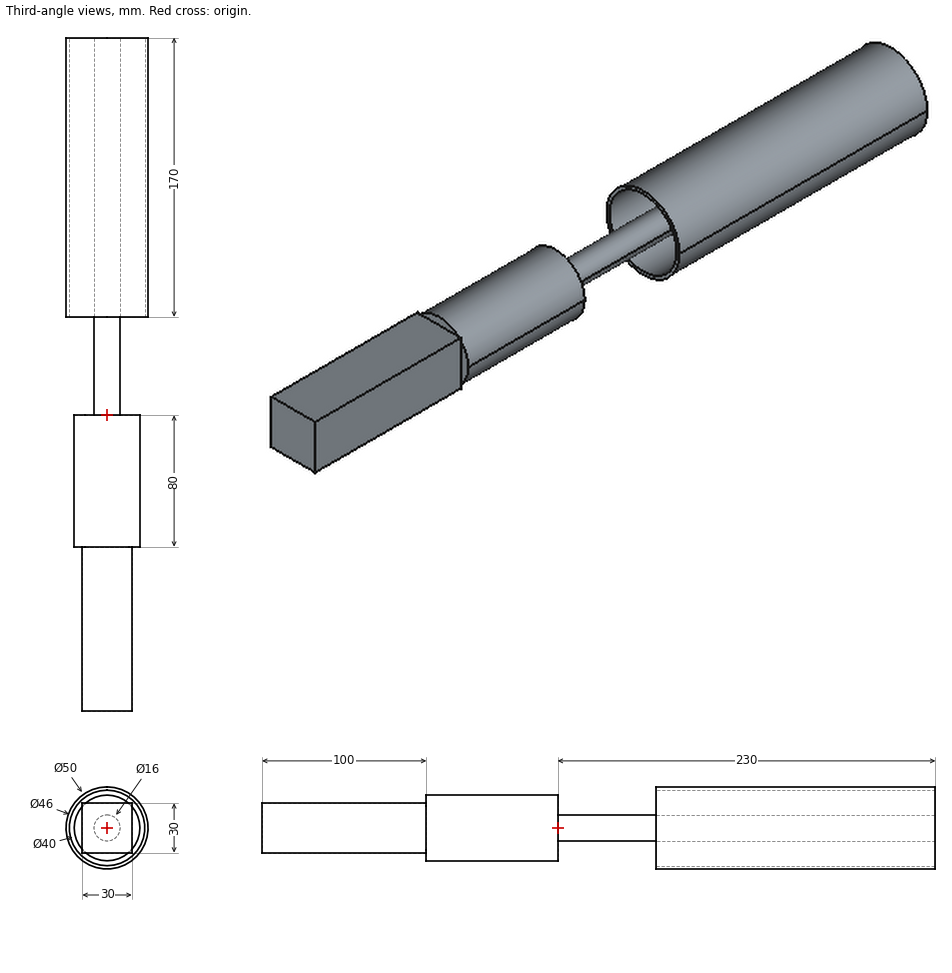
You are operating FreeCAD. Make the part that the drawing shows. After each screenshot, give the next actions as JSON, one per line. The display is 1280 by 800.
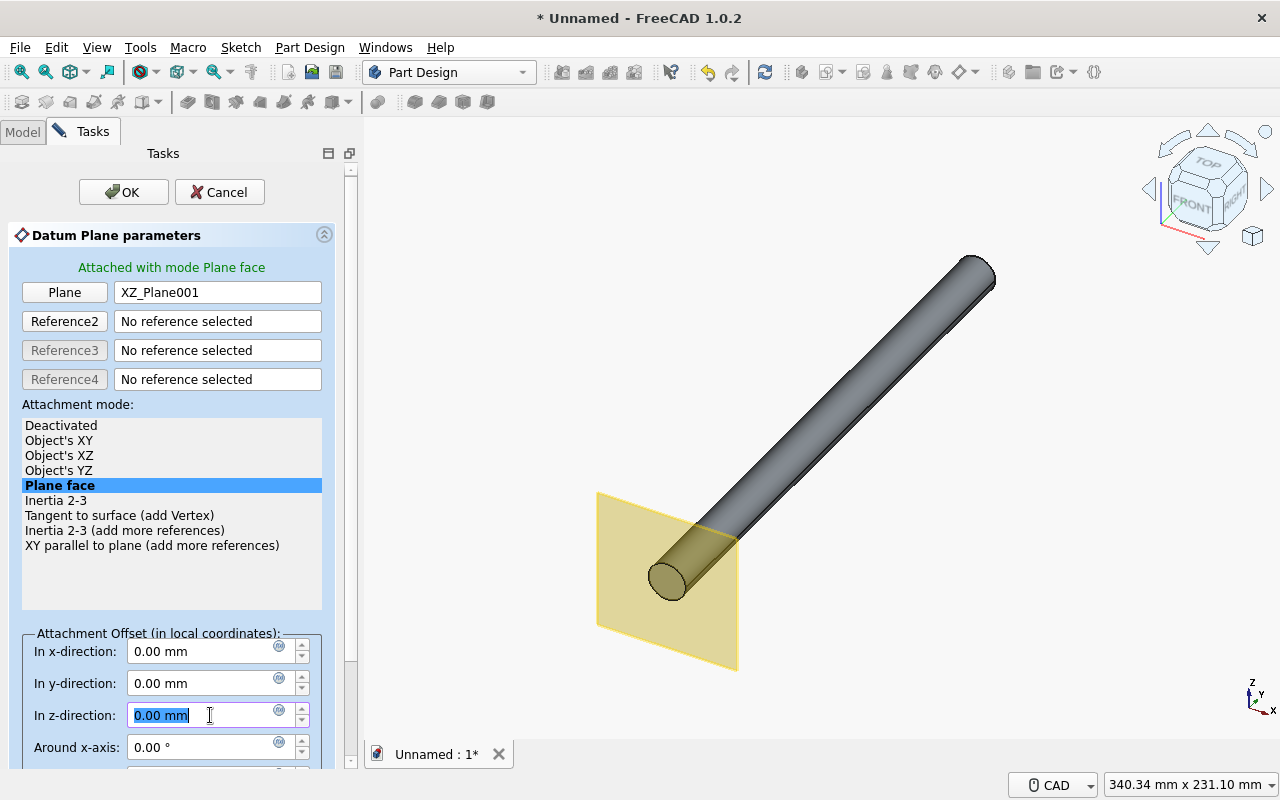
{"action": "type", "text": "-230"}
{"action": "key", "text": "Tab"}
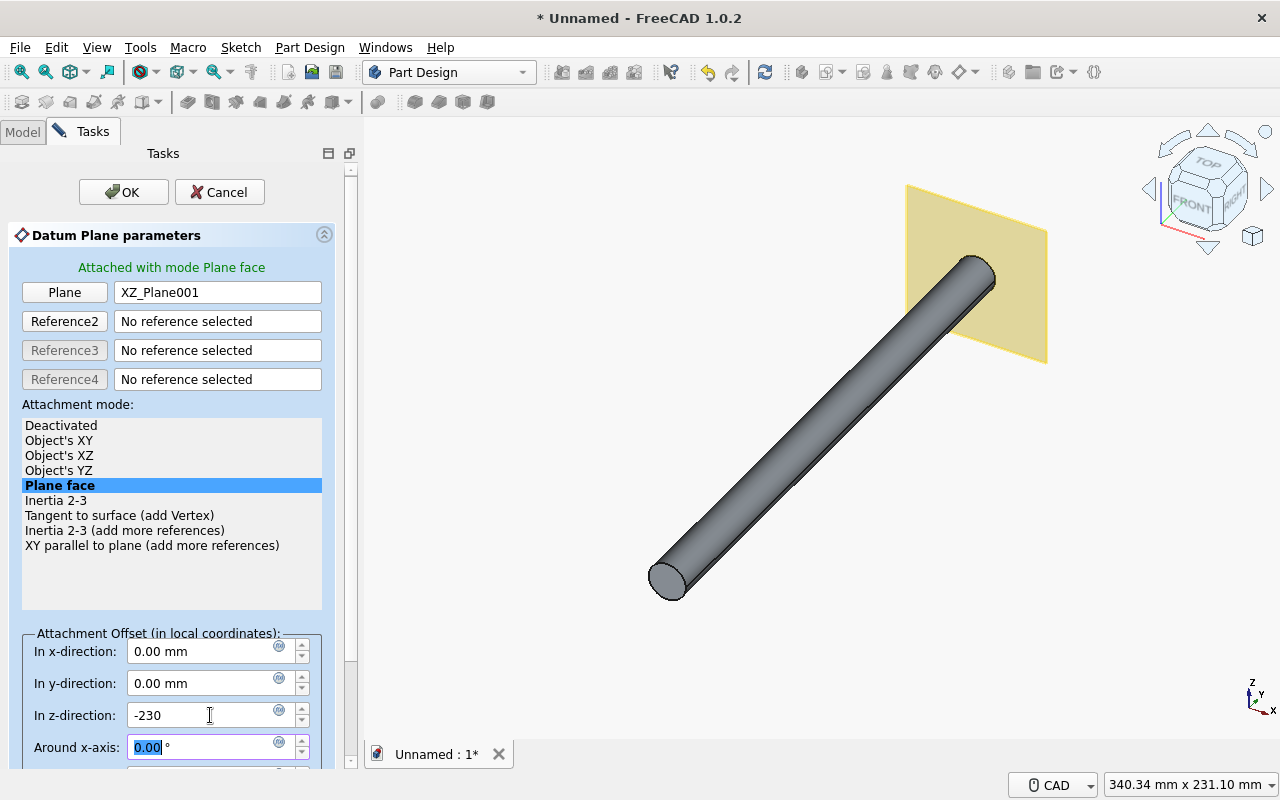
{"action": "left_click", "coordinate": [124, 192]}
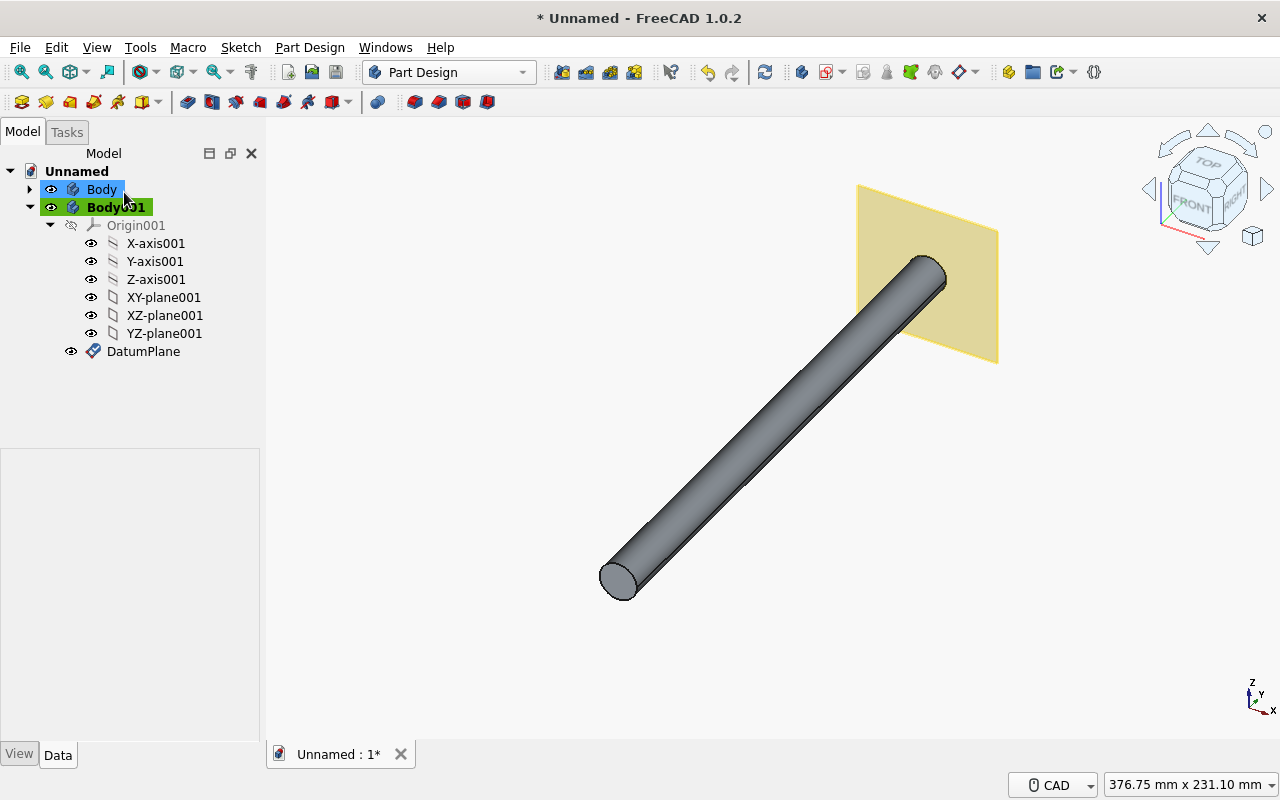
{"action": "left_click", "coordinate": [116, 351]}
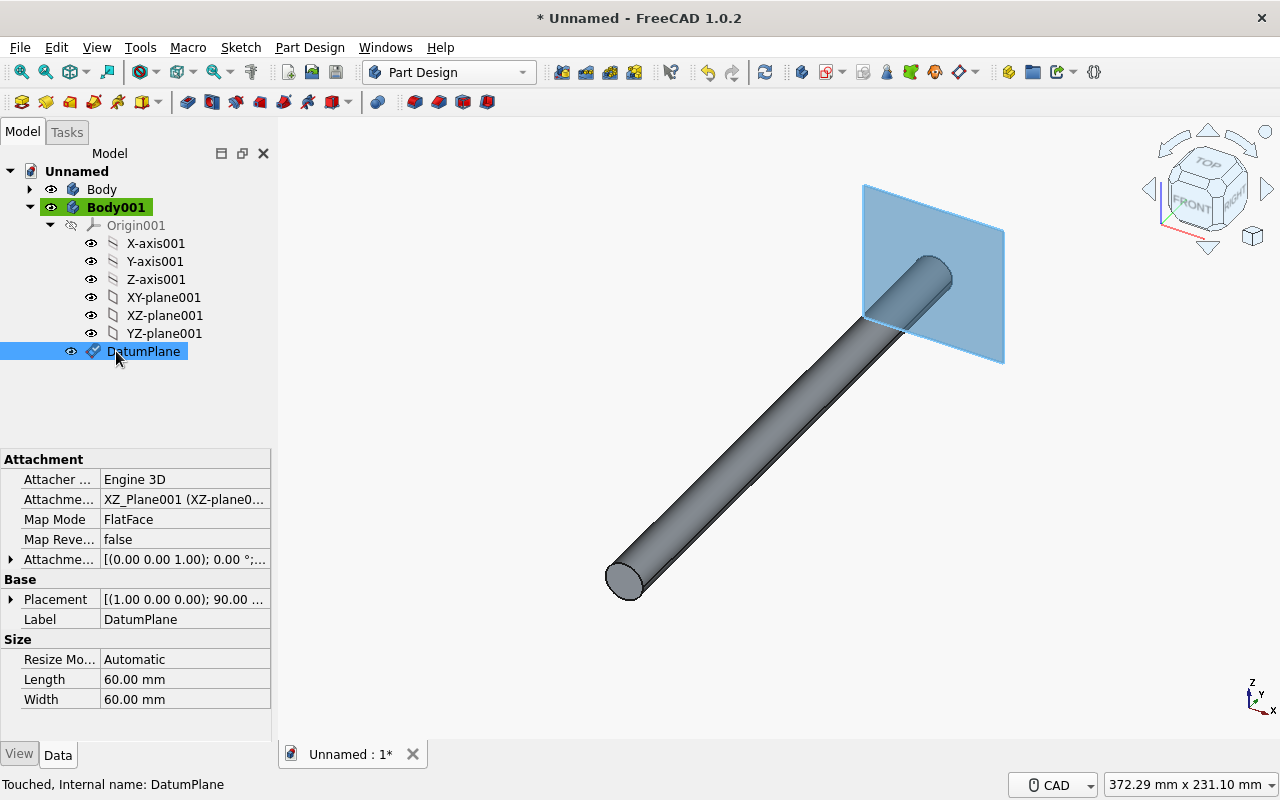
{"action": "left_click", "coordinate": [826, 72]}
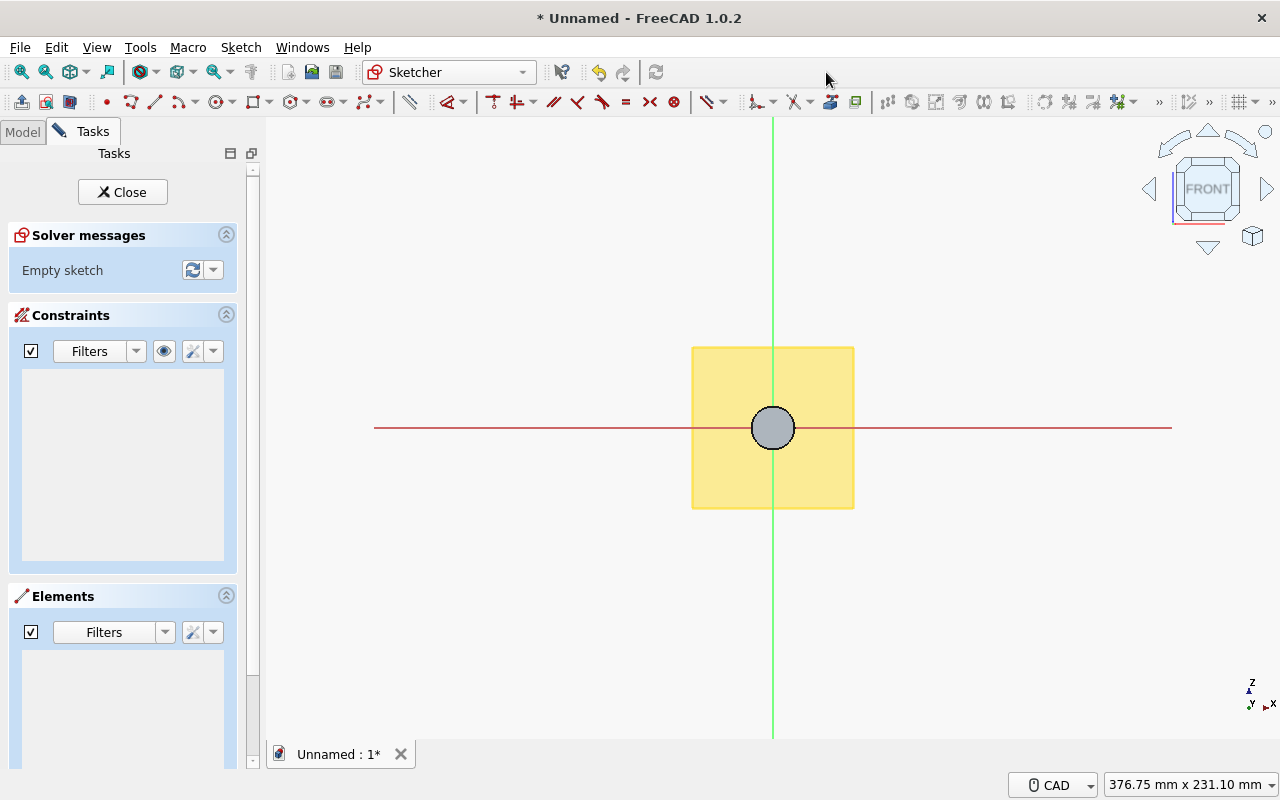
{"action": "scroll", "coordinate": [813, 428], "scroll_direction": "up", "scroll_amount": 5}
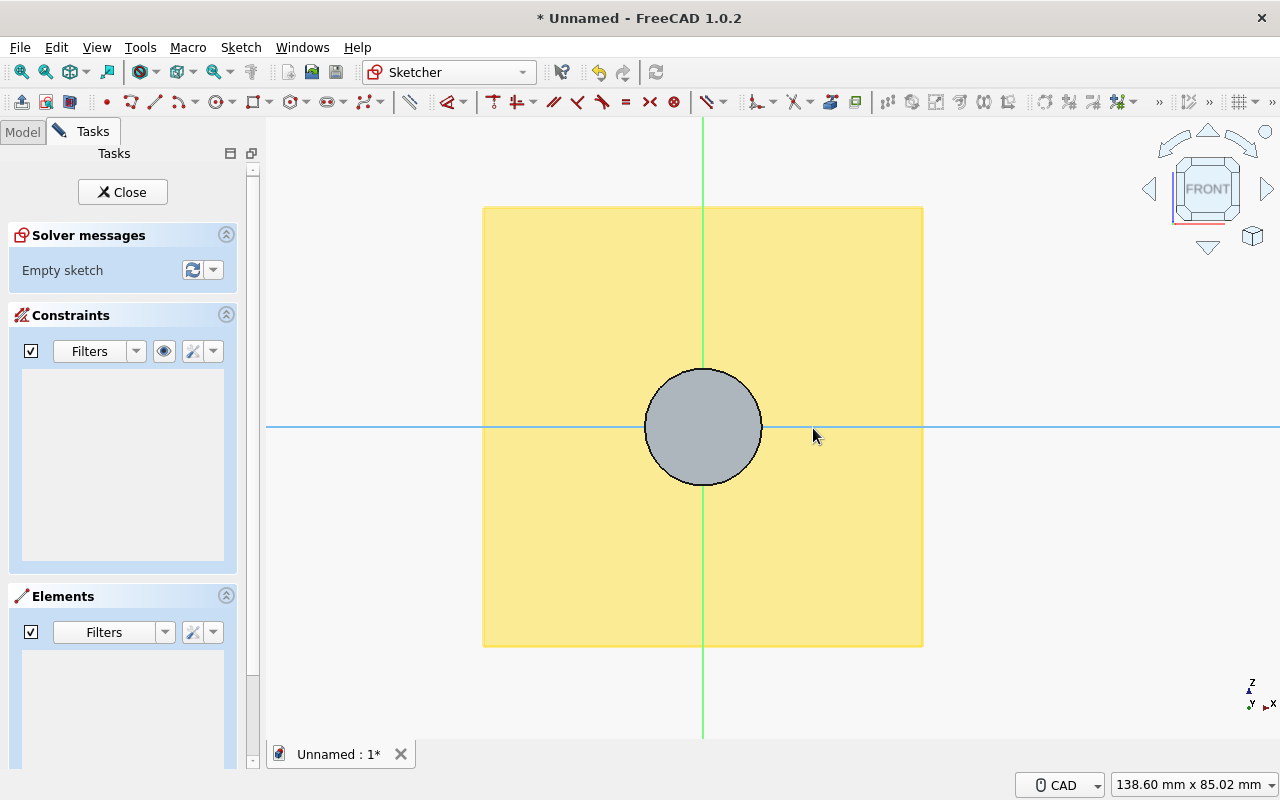
{"action": "left_click", "coordinate": [216, 102]}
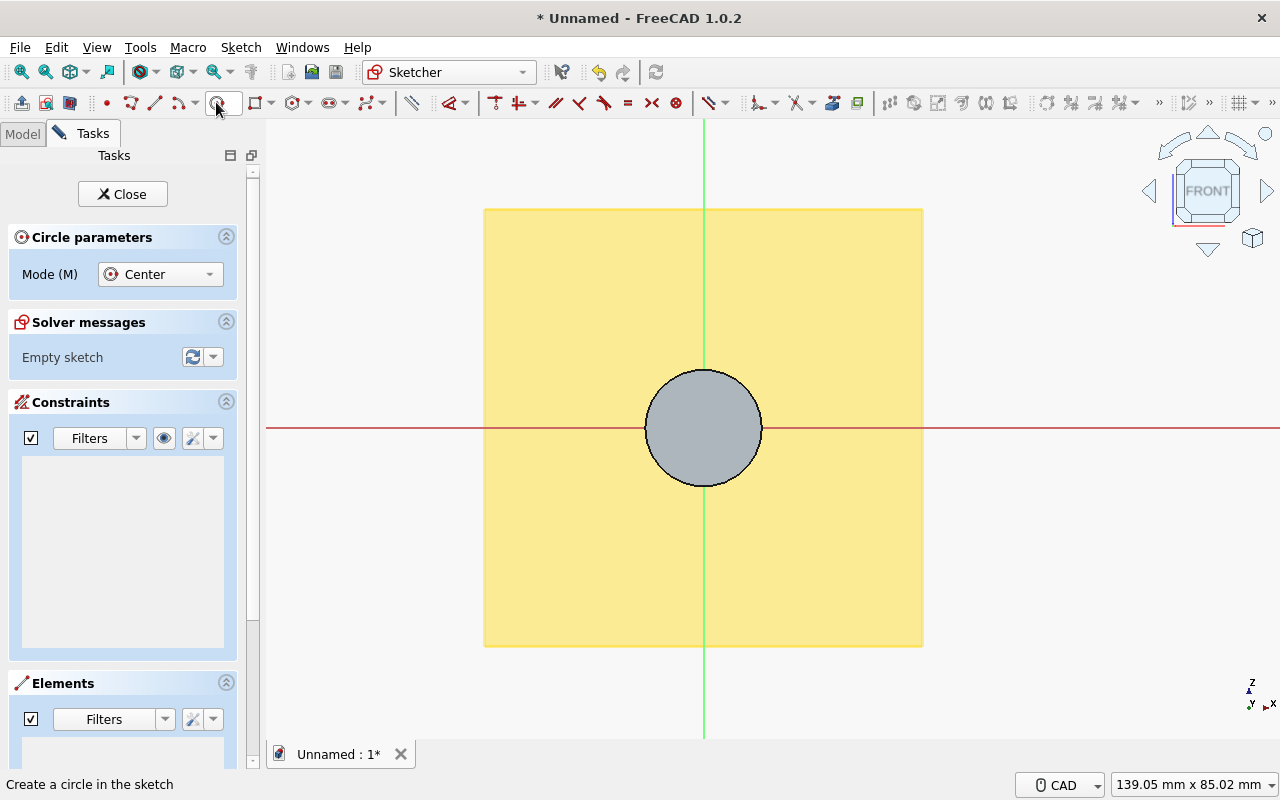
{"action": "left_click", "coordinate": [704, 428]}
{"action": "mouse_move", "coordinate": [832, 299]}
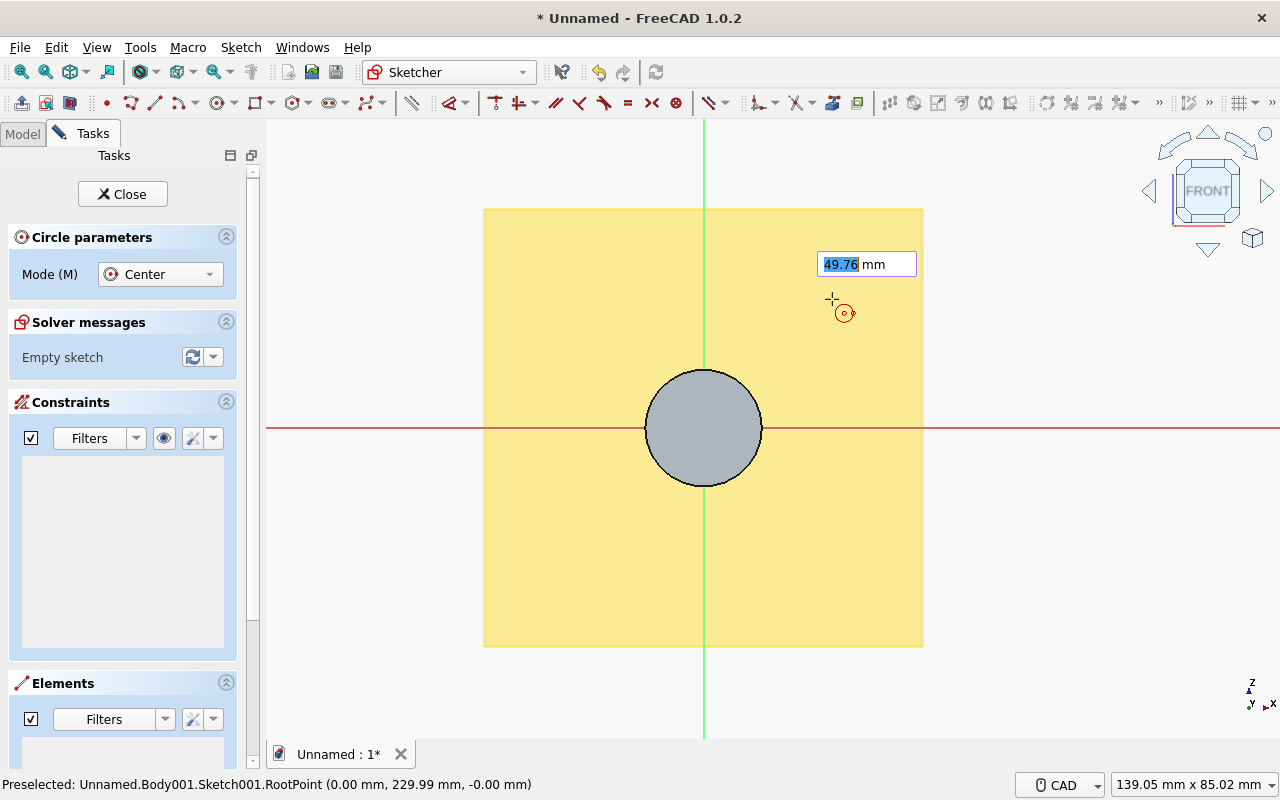
{"action": "type", "text": "50"}
{"action": "key", "text": "Return"}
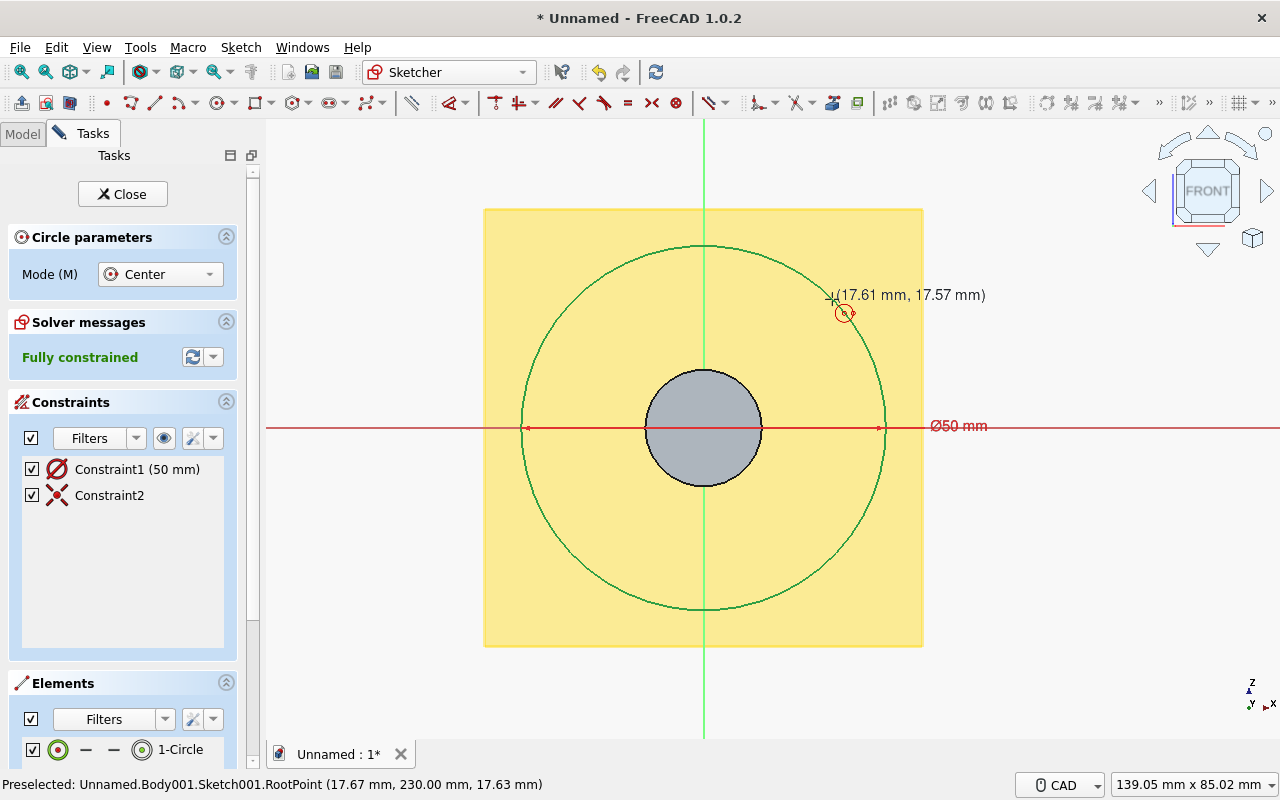
{"action": "left_click", "coordinate": [704, 428]}
{"action": "mouse_move", "coordinate": [822, 310]}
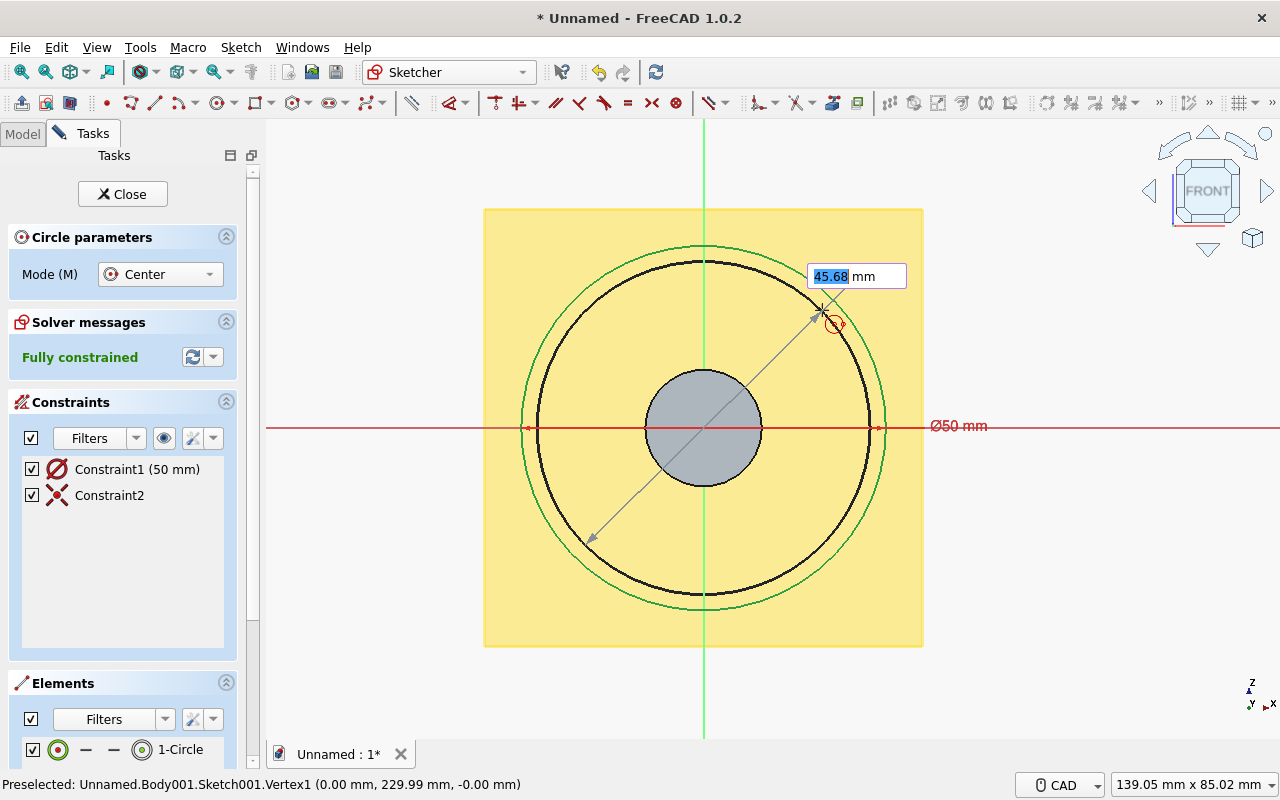
{"action": "type", "text": "46"}
{"action": "key", "text": "Return"}
{"action": "key", "text": "Escape"}